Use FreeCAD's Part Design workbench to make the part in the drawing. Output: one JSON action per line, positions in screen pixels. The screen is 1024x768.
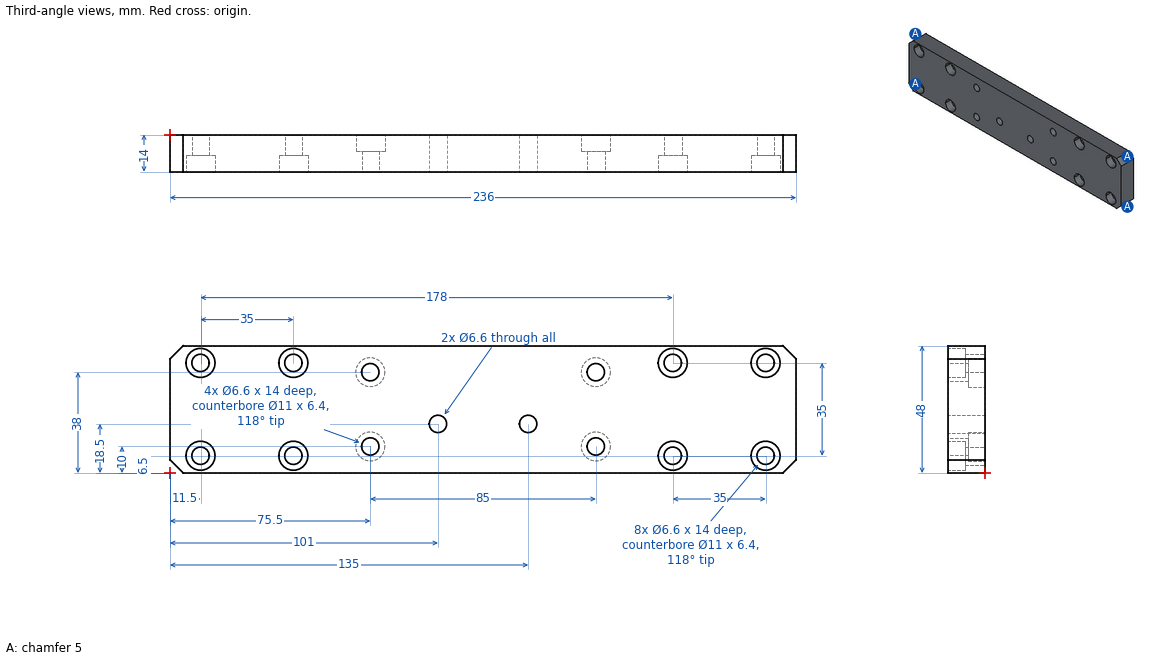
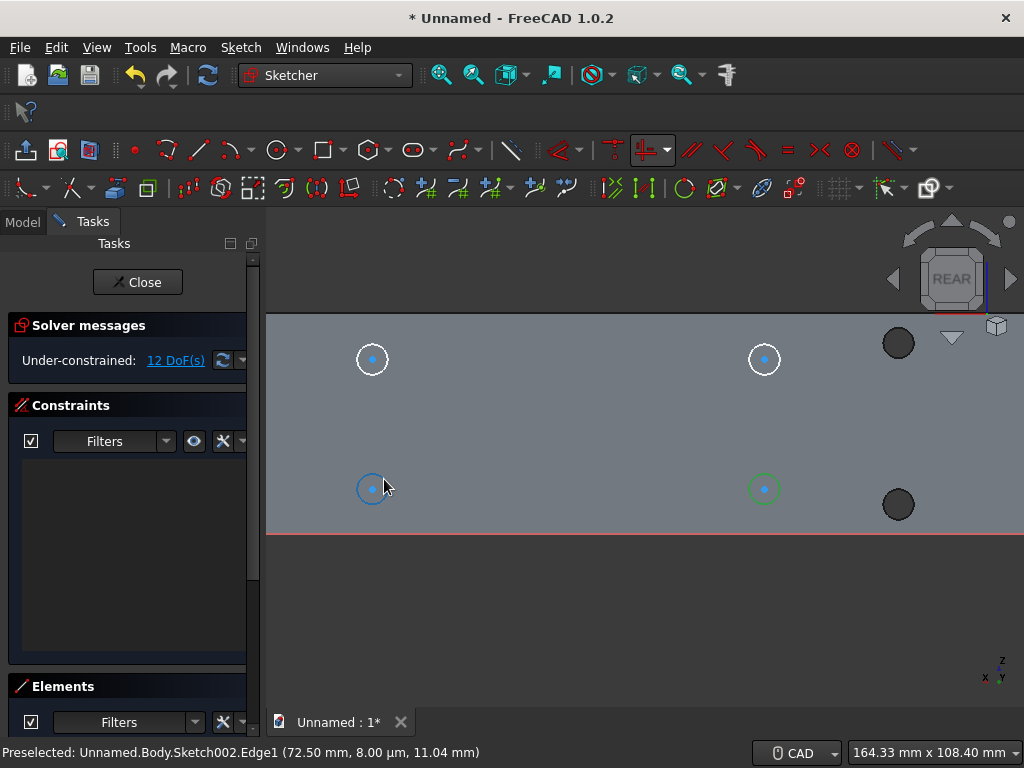
{"action": "left_click", "coordinate": [383, 478]}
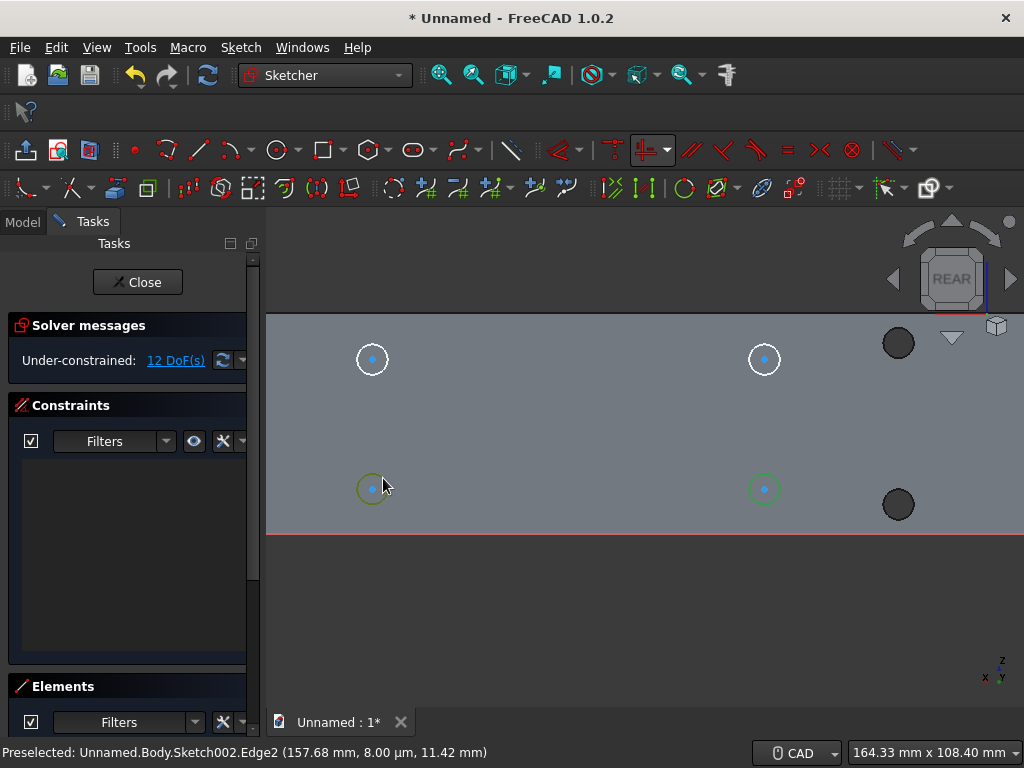
{"action": "left_click", "coordinate": [775, 349]}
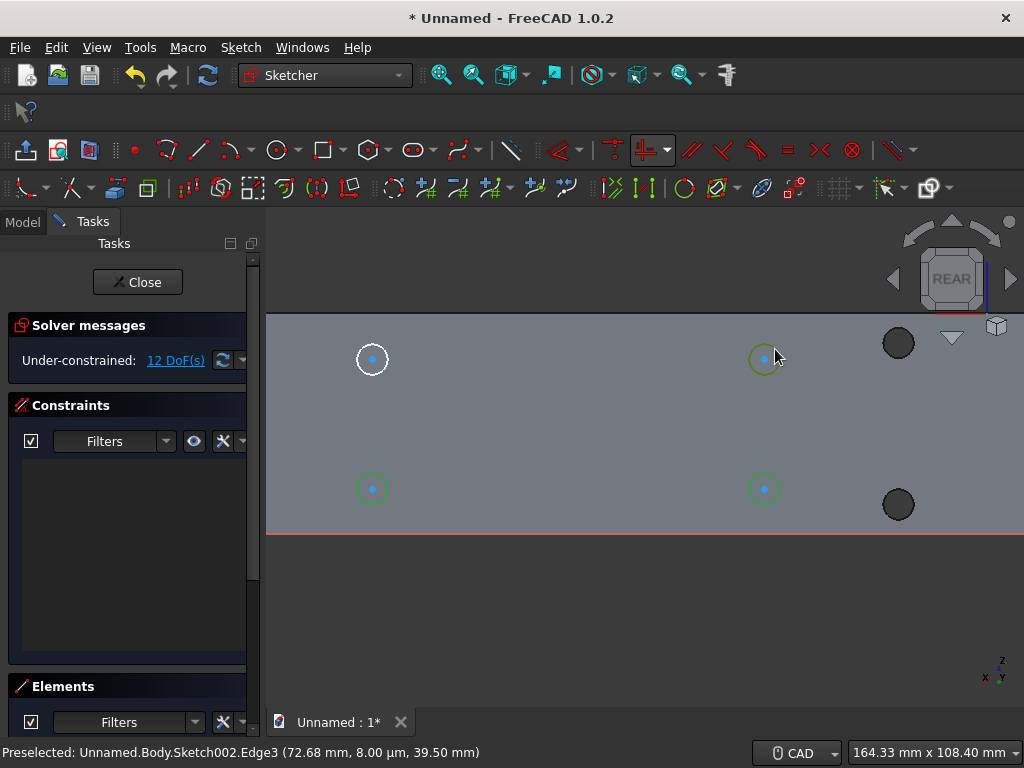
{"action": "left_click", "coordinate": [383, 349]}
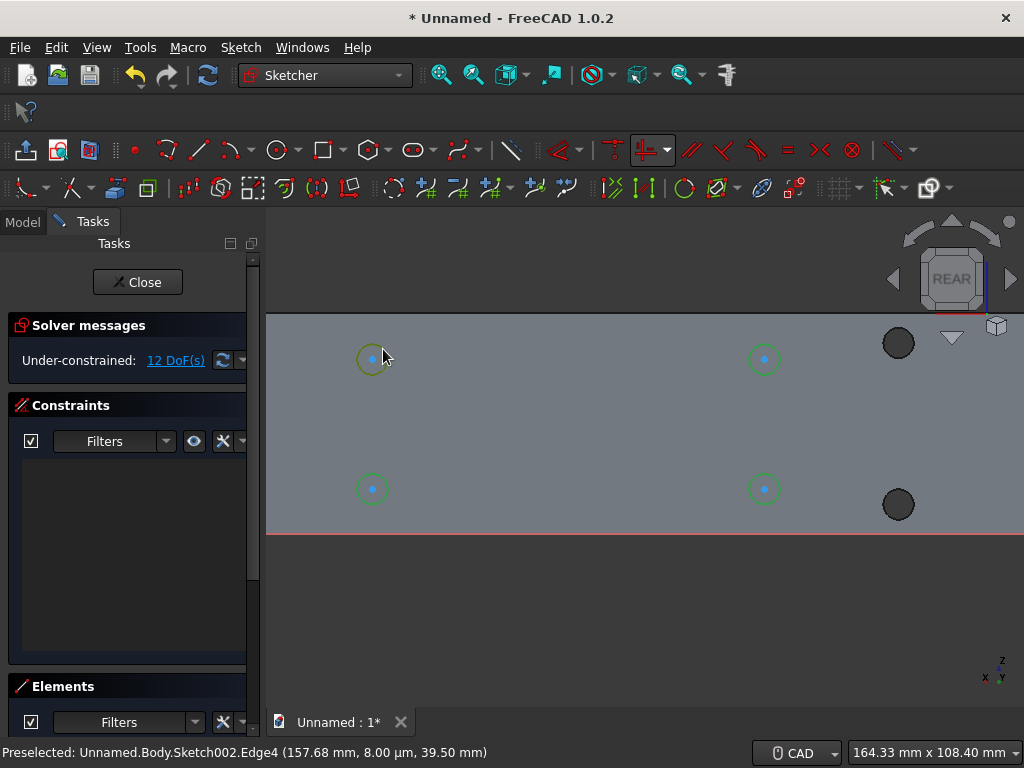
{"action": "left_click", "coordinate": [788, 150]}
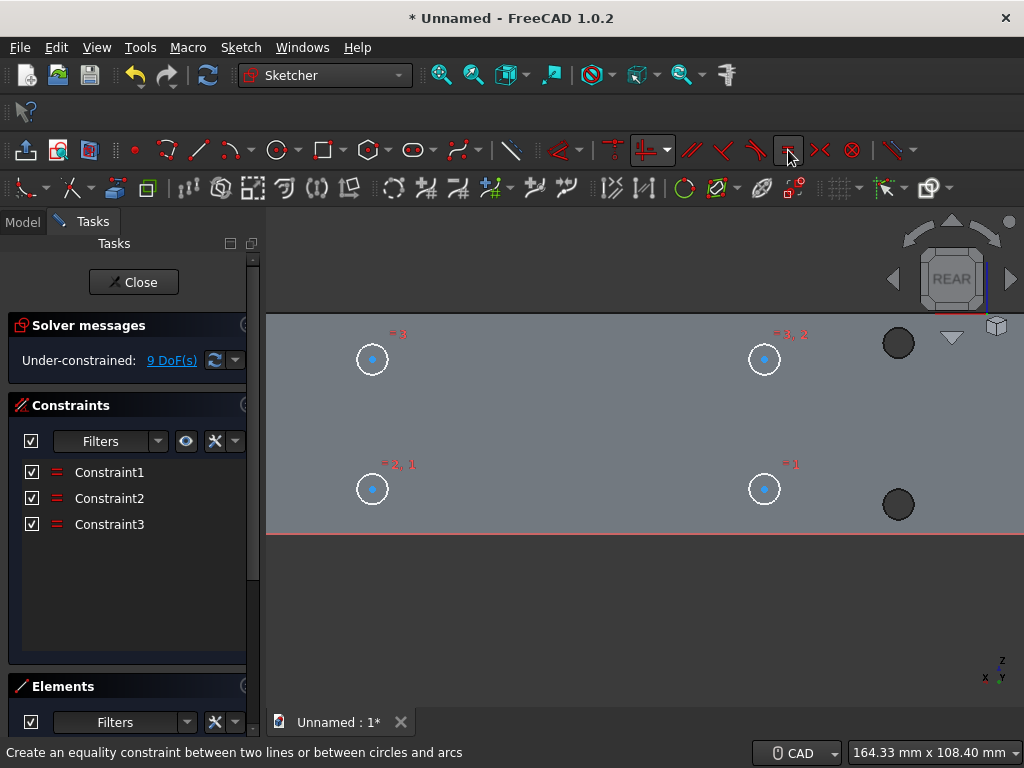
{"action": "left_click", "coordinate": [765, 489]}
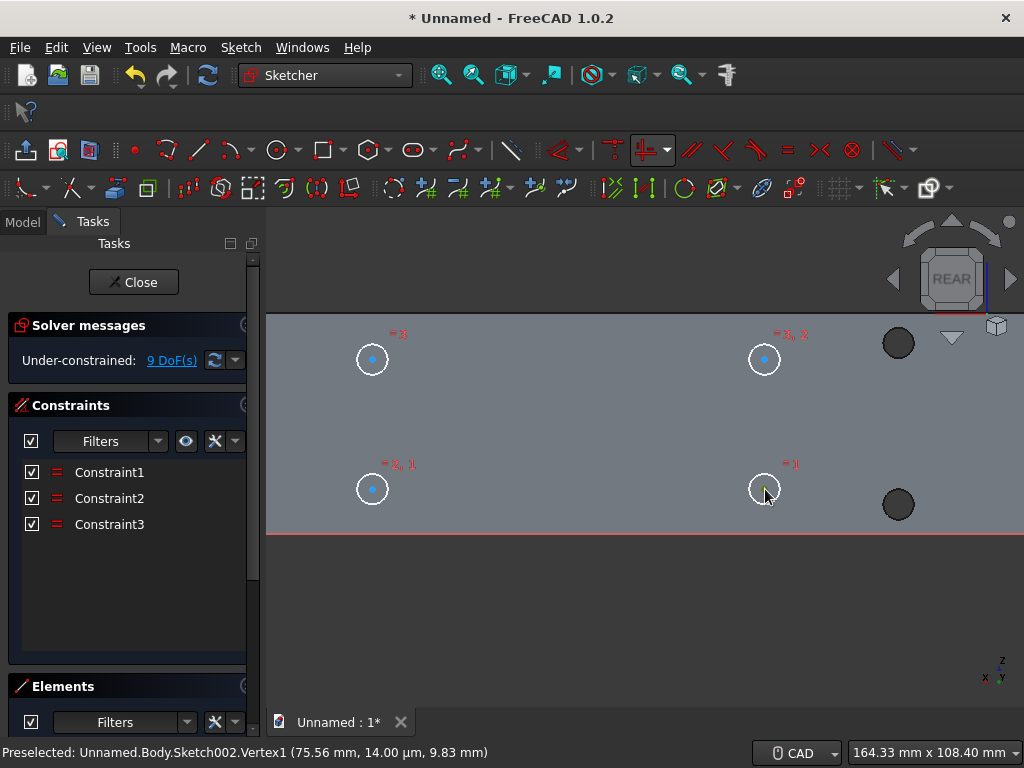
{"action": "left_click", "coordinate": [372, 489]}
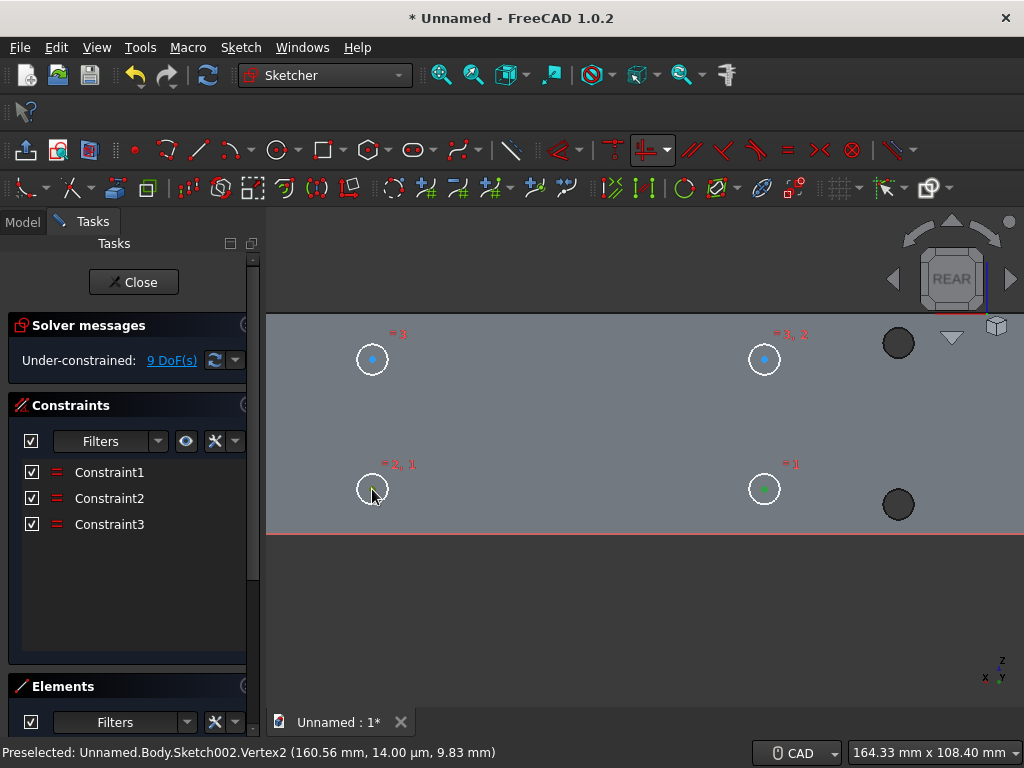
{"action": "left_click", "coordinate": [670, 150]}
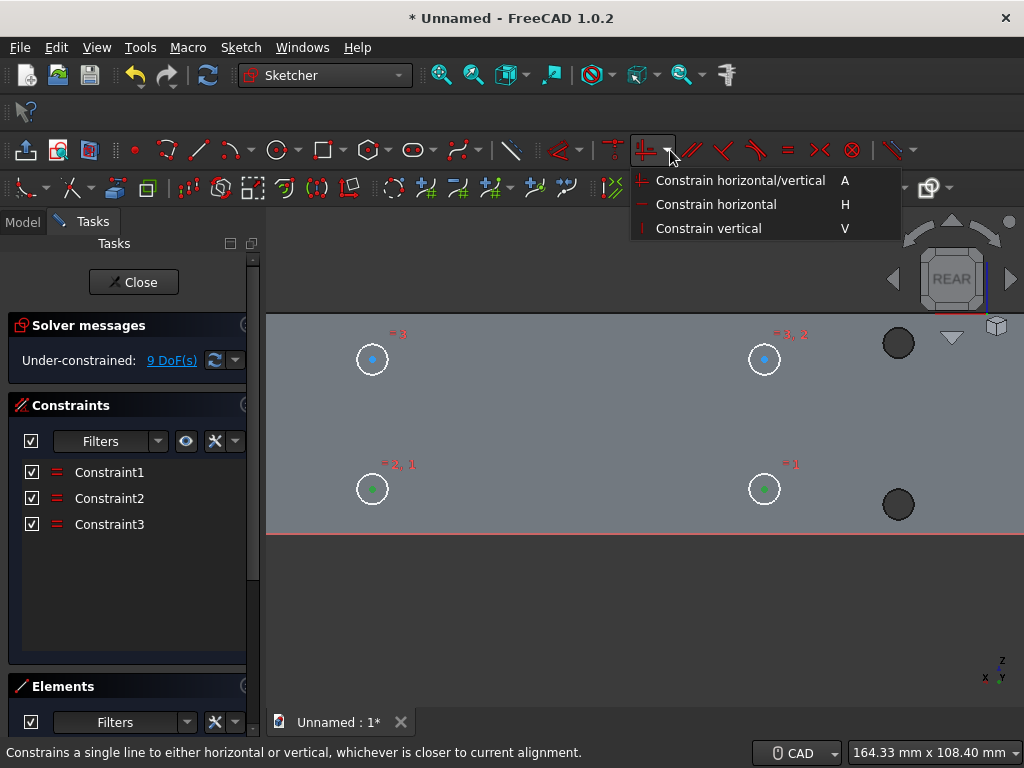
{"action": "left_click", "coordinate": [766, 204]}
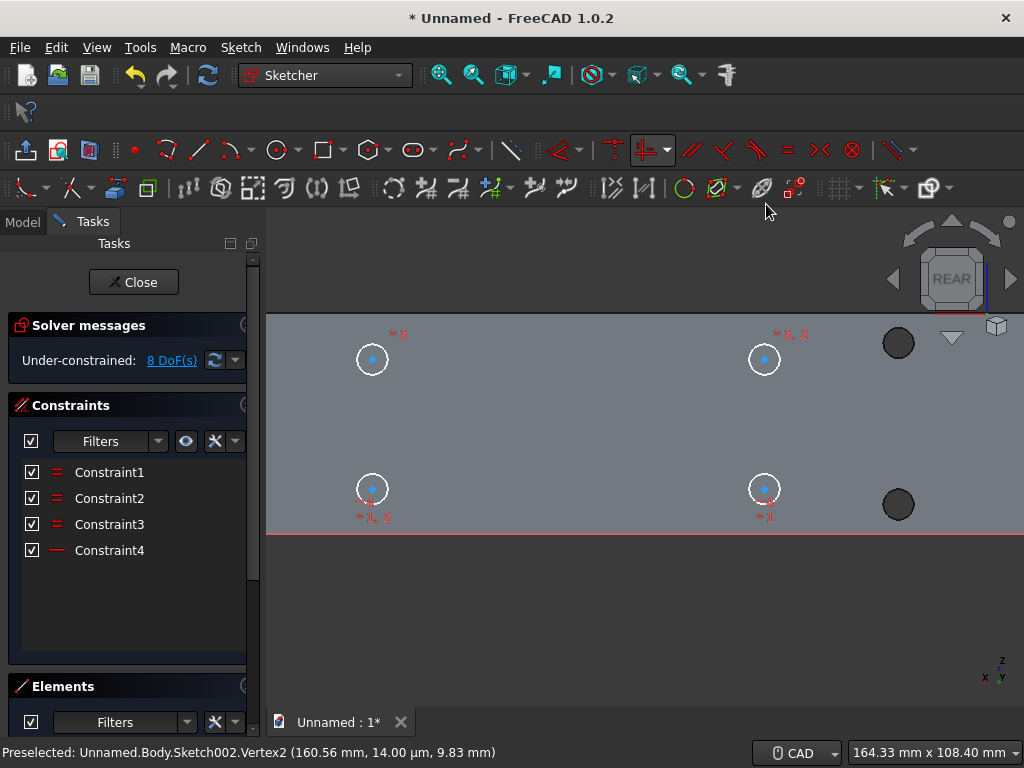
{"action": "left_click", "coordinate": [765, 489]}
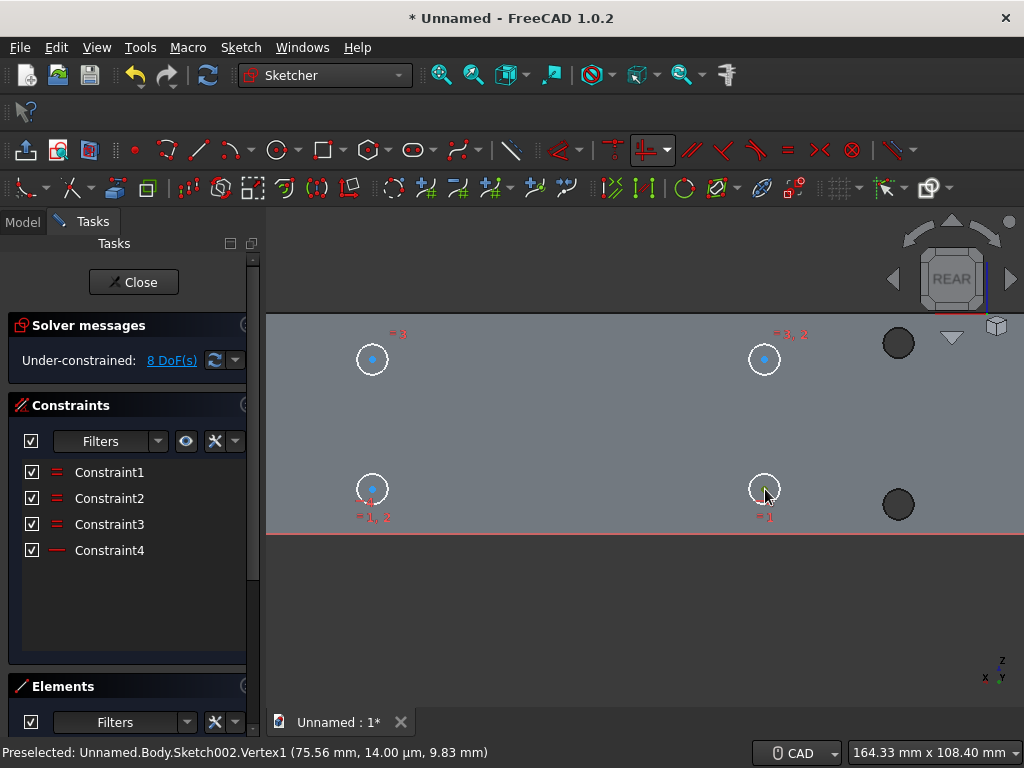
{"action": "left_click", "coordinate": [765, 360]}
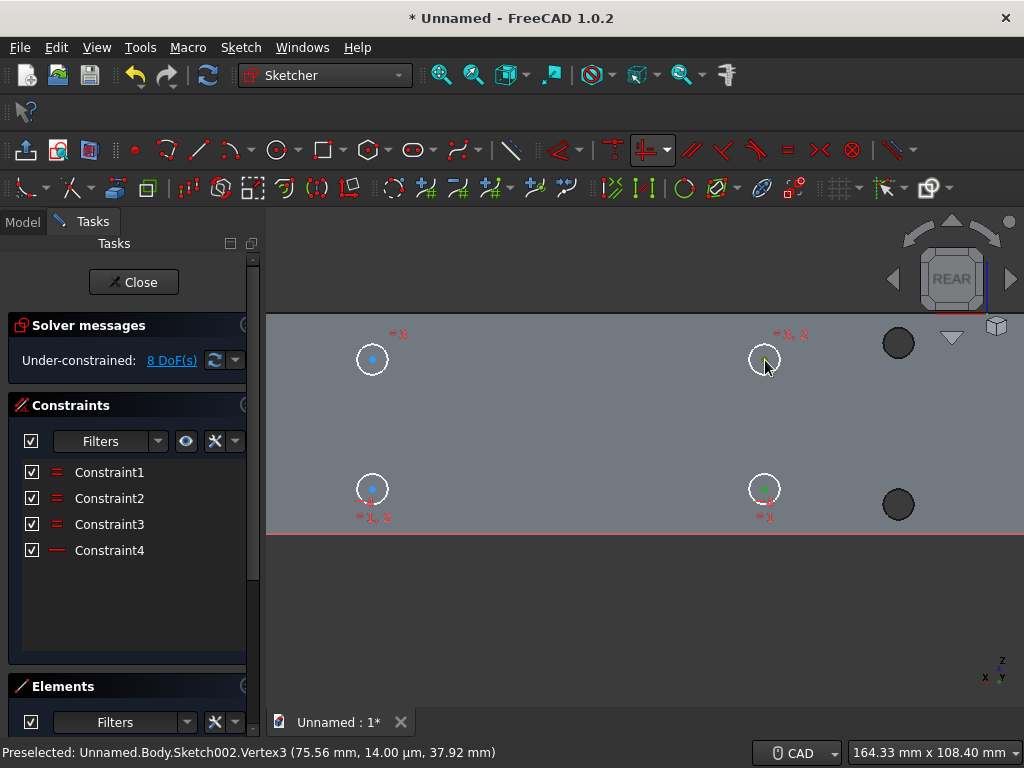
{"action": "left_click", "coordinate": [670, 150]}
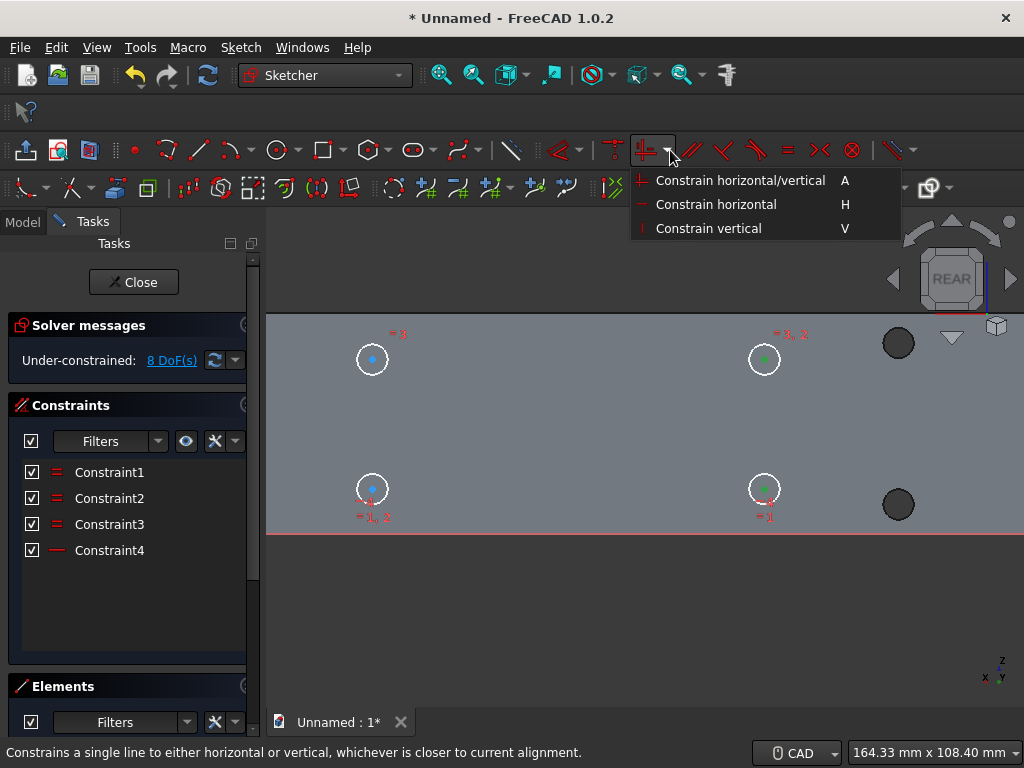
{"action": "left_click", "coordinate": [766, 228]}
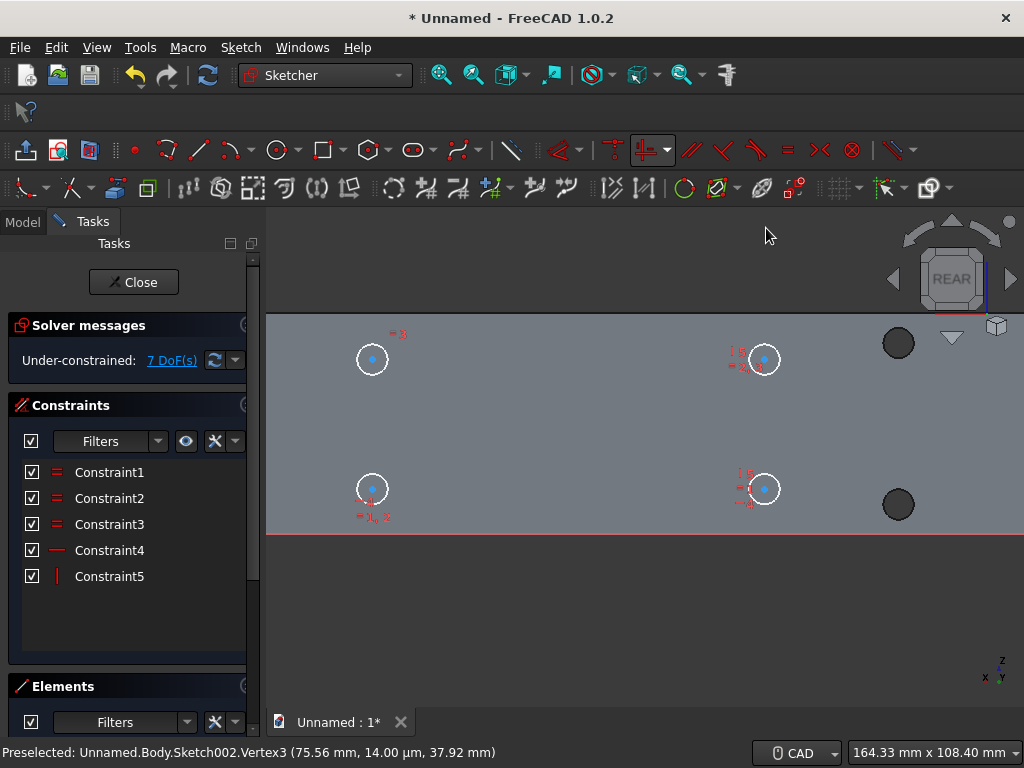
{"action": "left_click", "coordinate": [372, 489]}